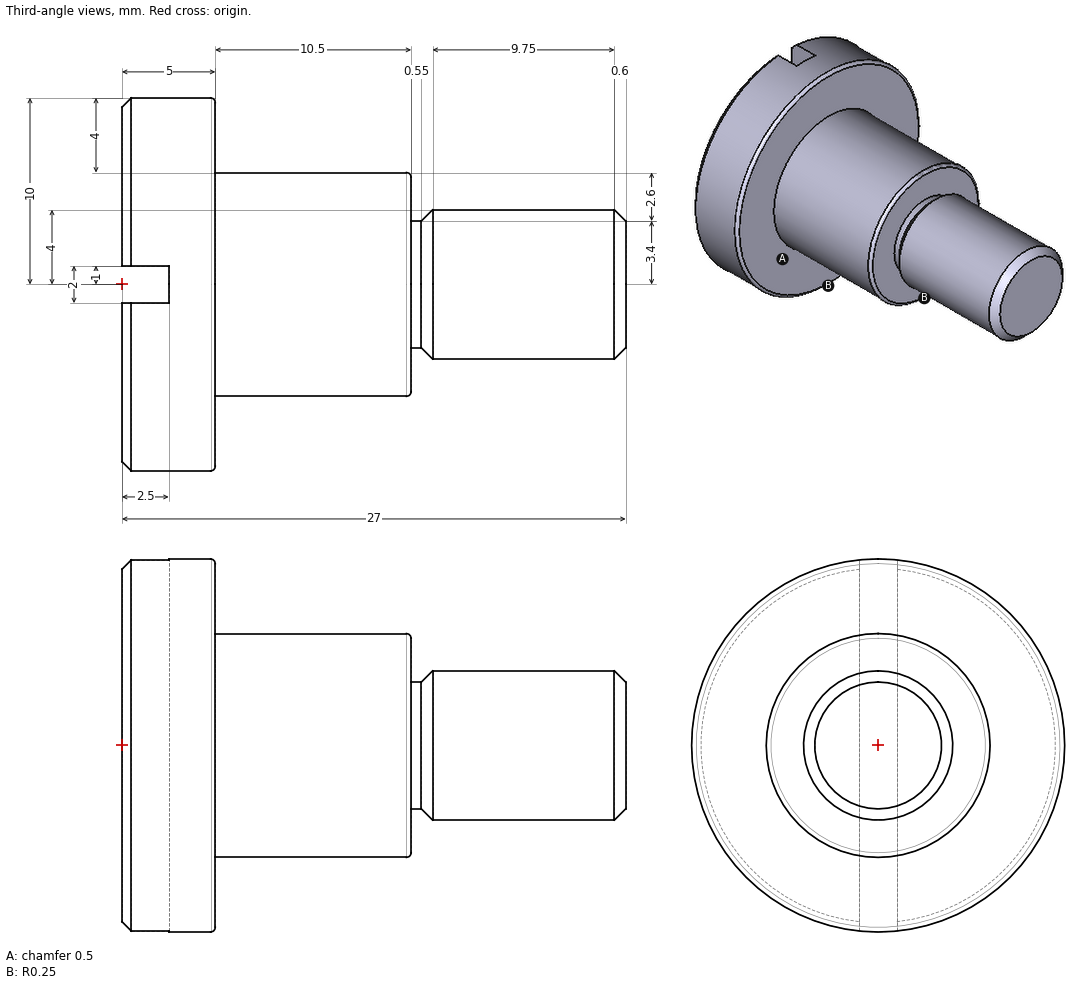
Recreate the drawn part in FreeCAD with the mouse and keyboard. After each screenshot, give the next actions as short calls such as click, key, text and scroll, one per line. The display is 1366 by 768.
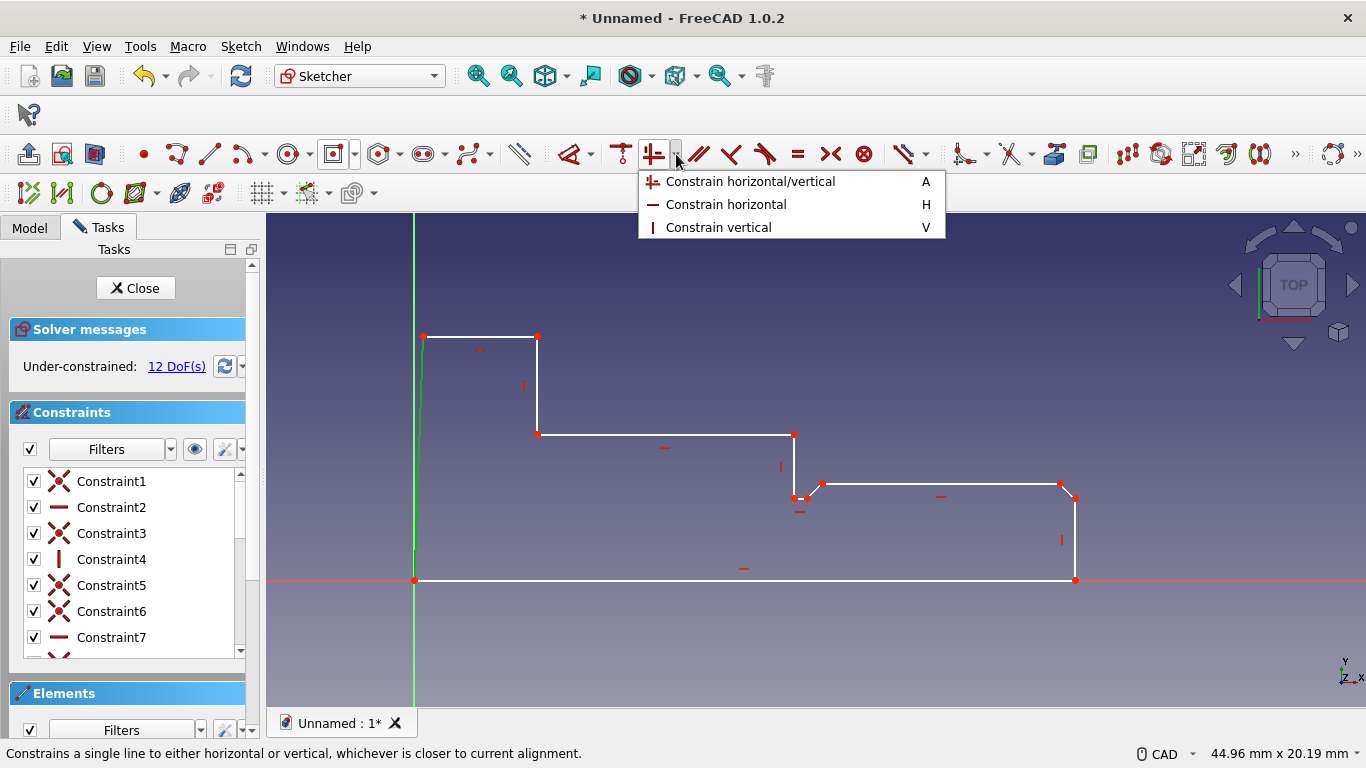
click(792, 228)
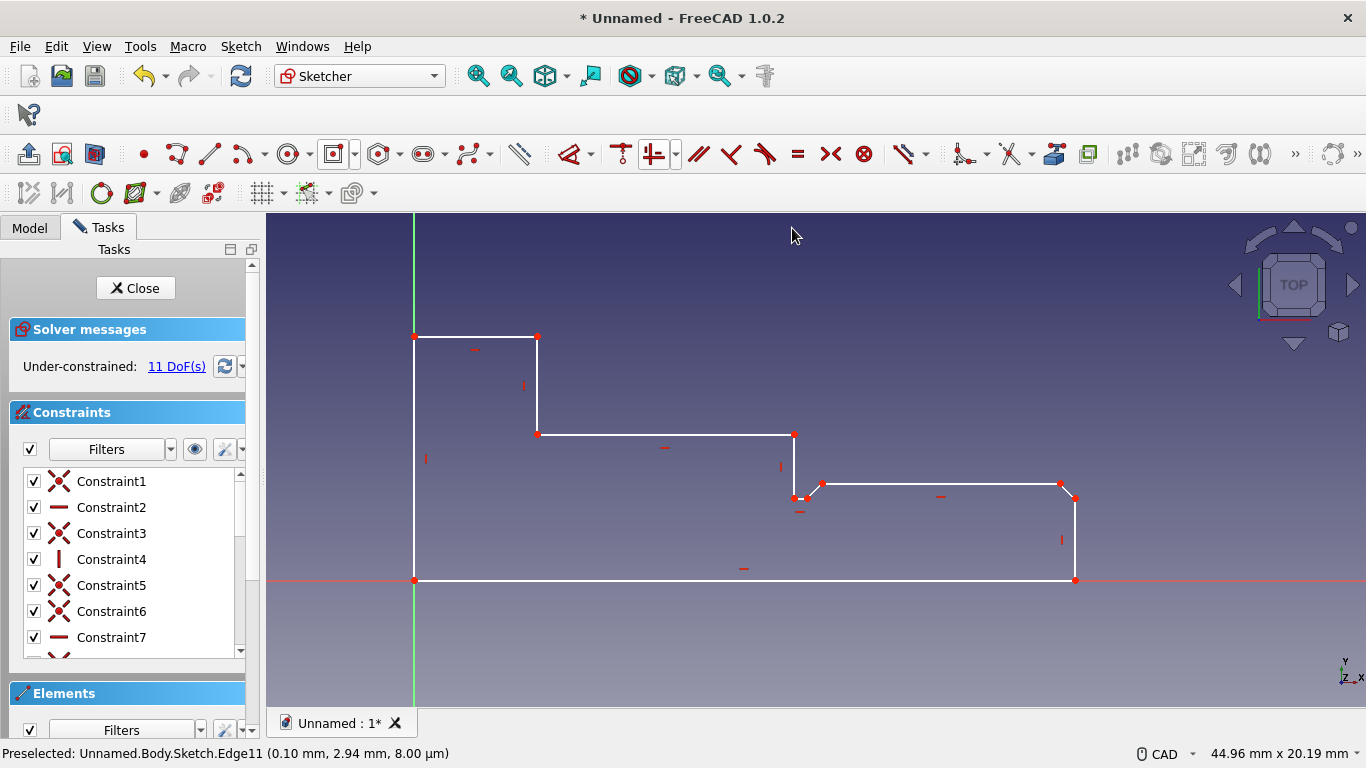
key(d)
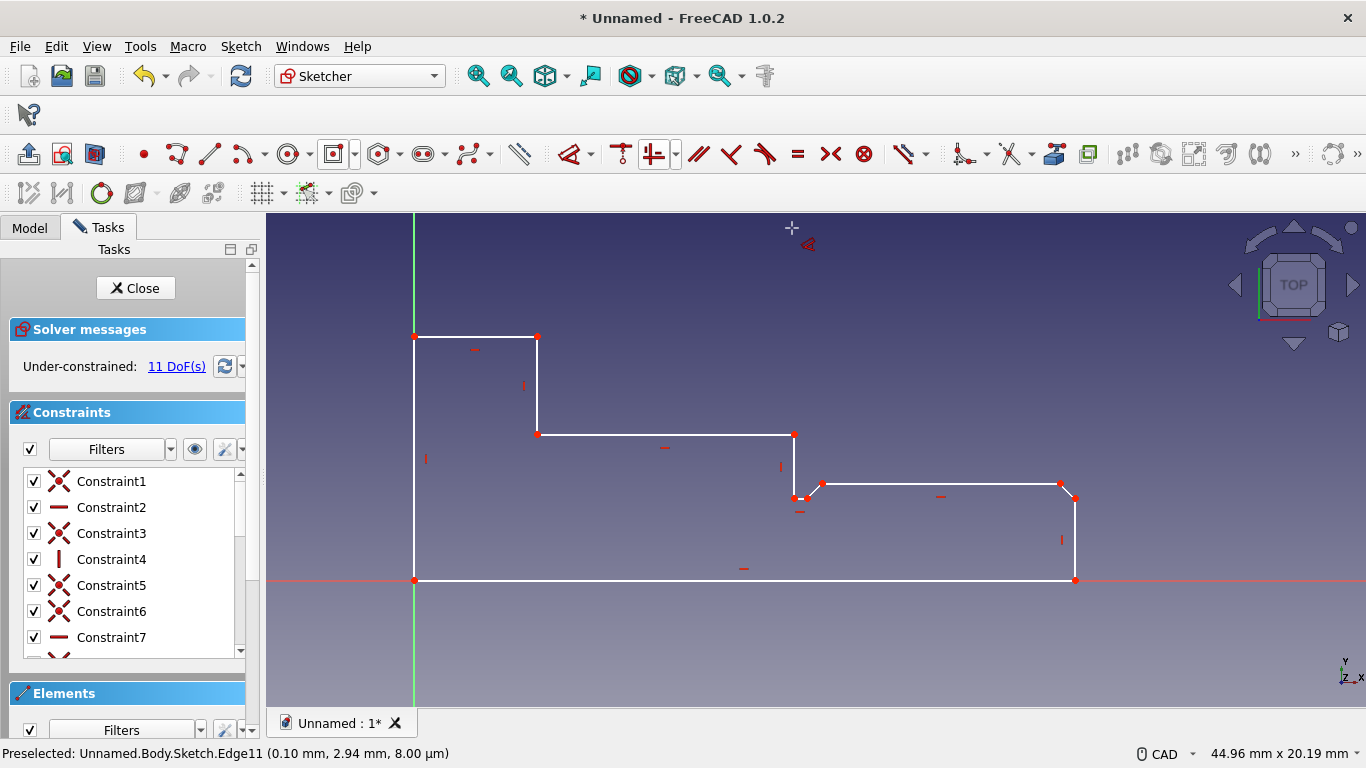
click(537, 406)
click(503, 386)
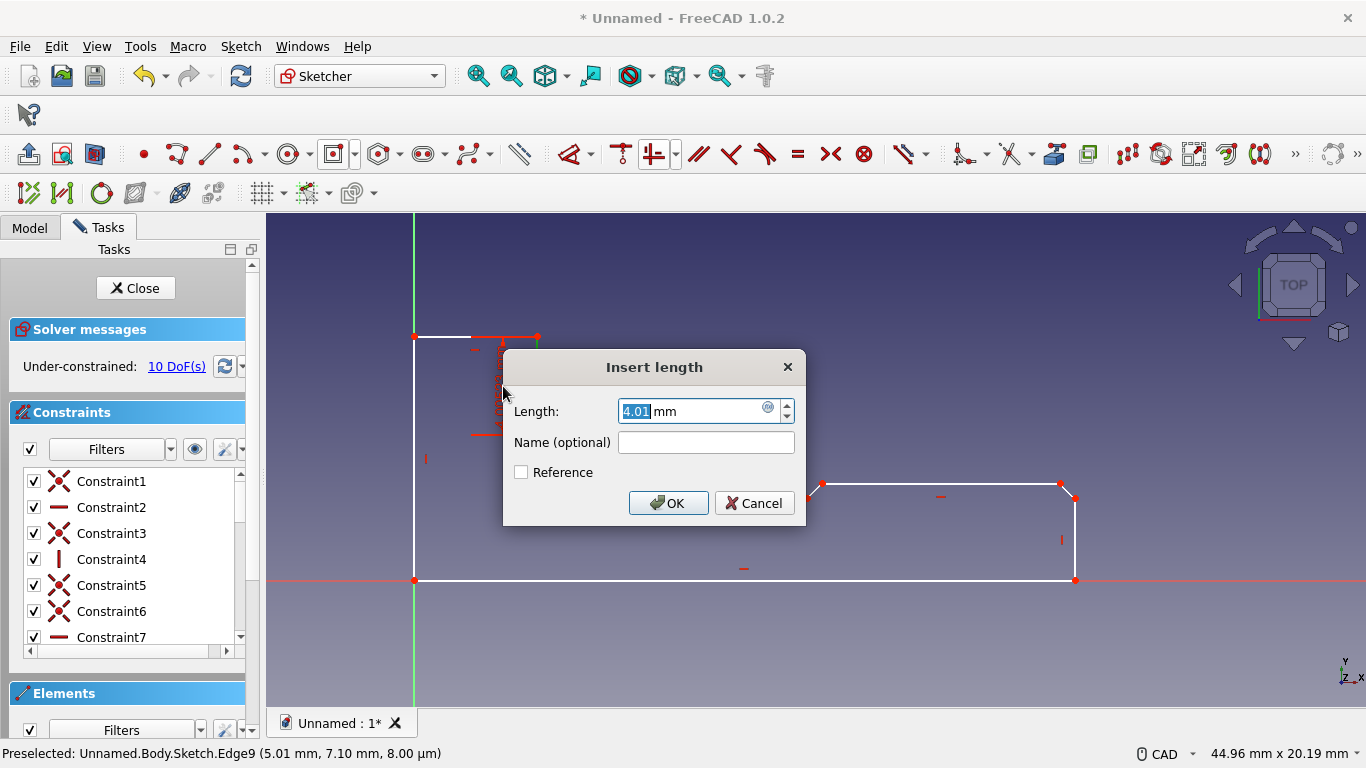
text(4)
key(Return)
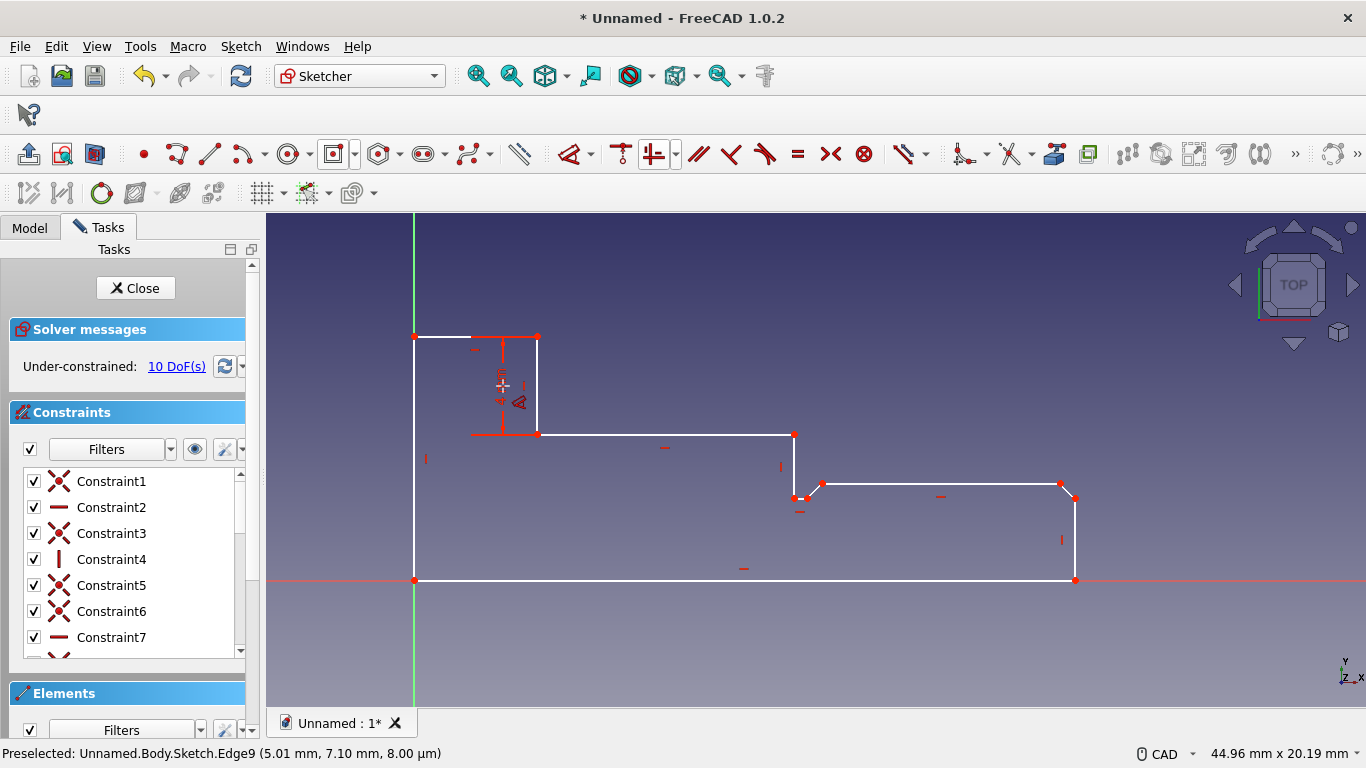
click(500, 337)
click(476, 303)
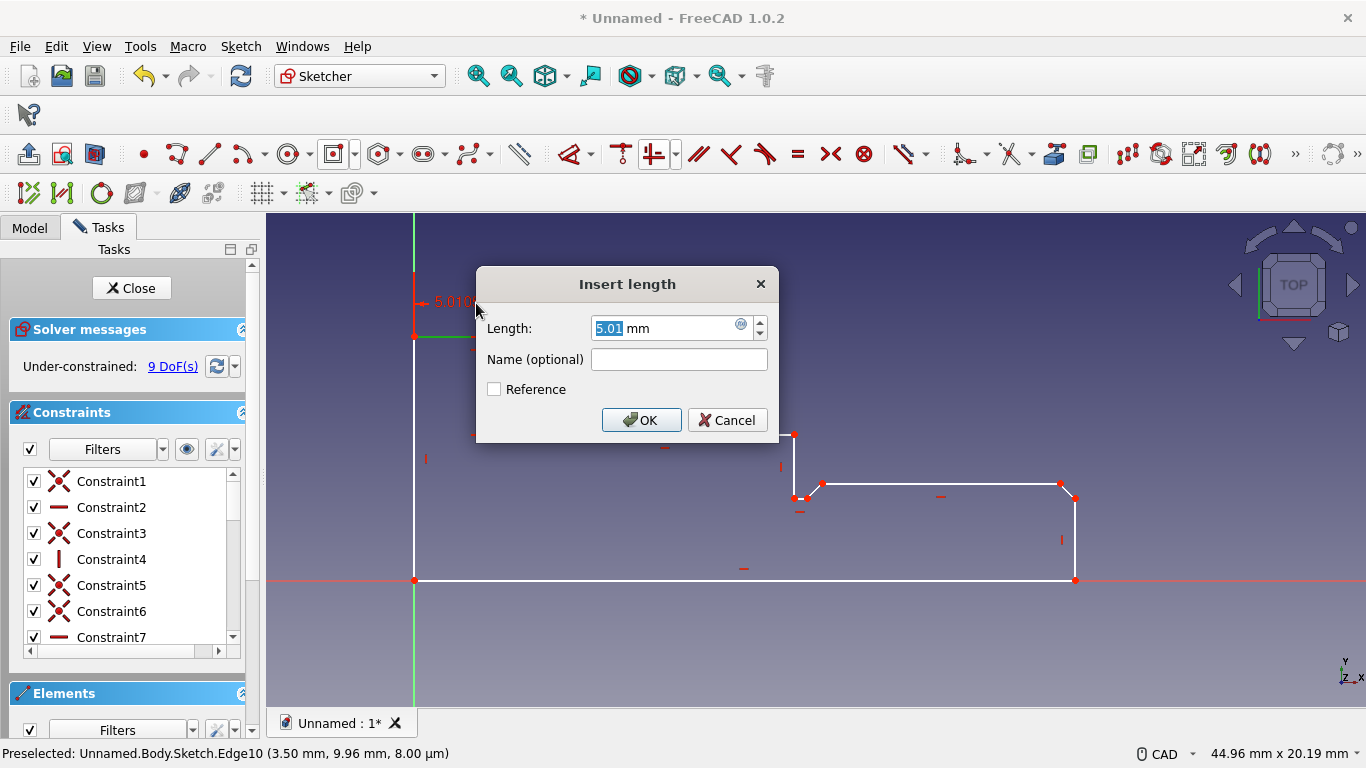
text(5)
key(Return)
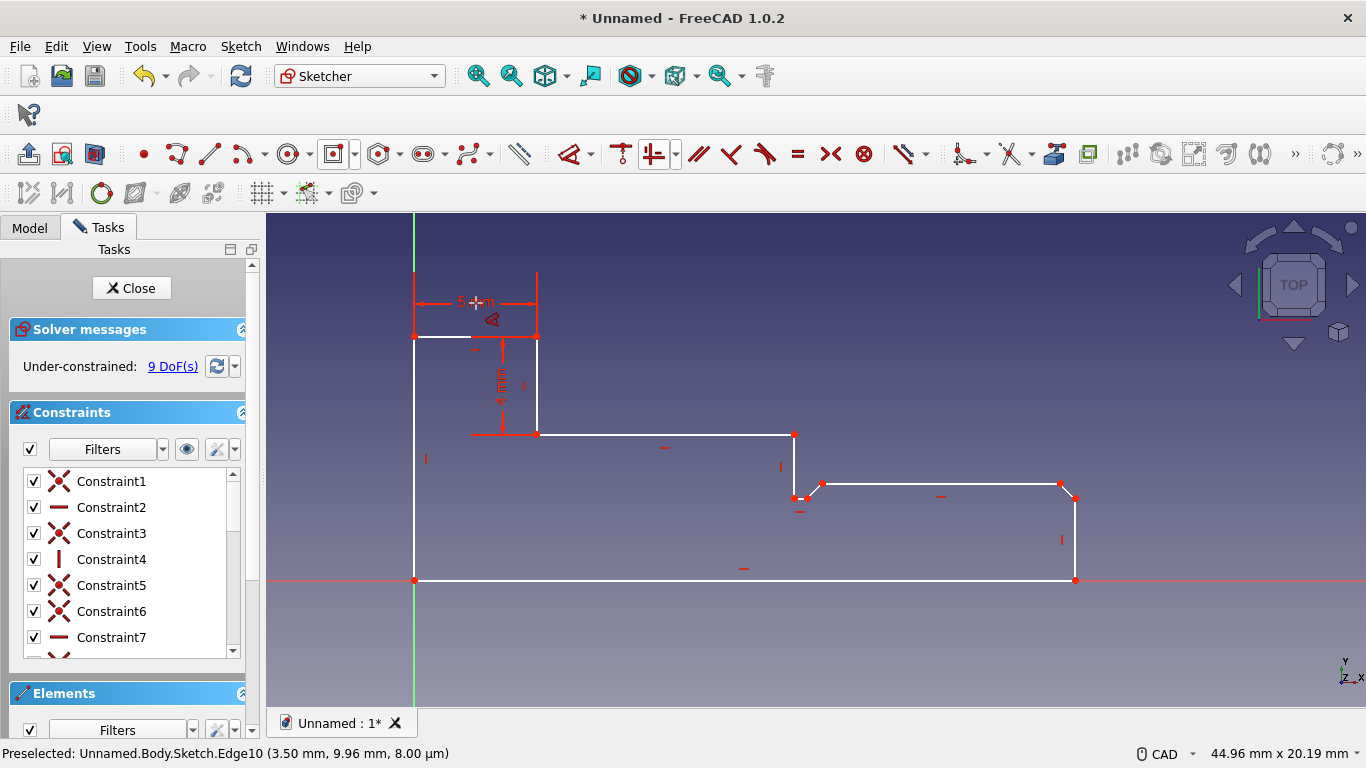
click(613, 581)
click(745, 615)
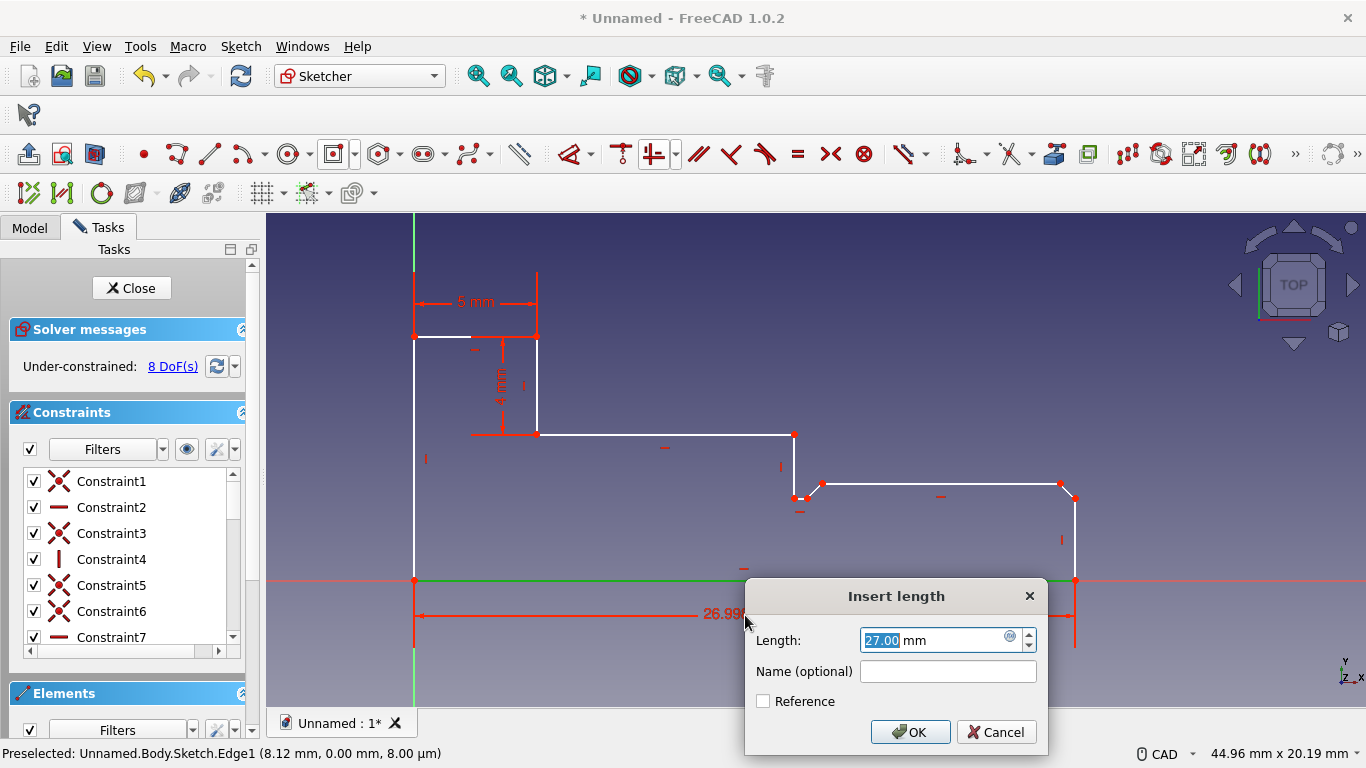
text(27)
key(Return)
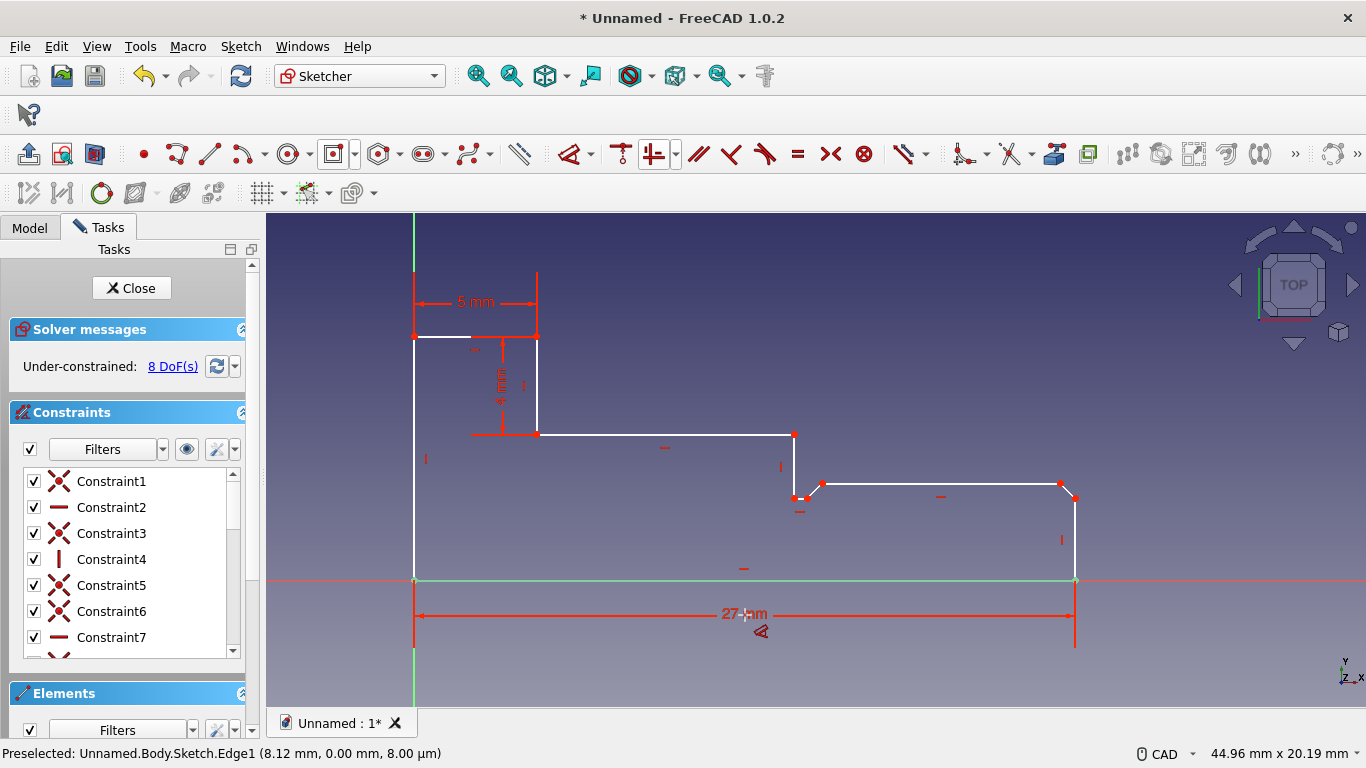
click(414, 410)
click(380, 459)